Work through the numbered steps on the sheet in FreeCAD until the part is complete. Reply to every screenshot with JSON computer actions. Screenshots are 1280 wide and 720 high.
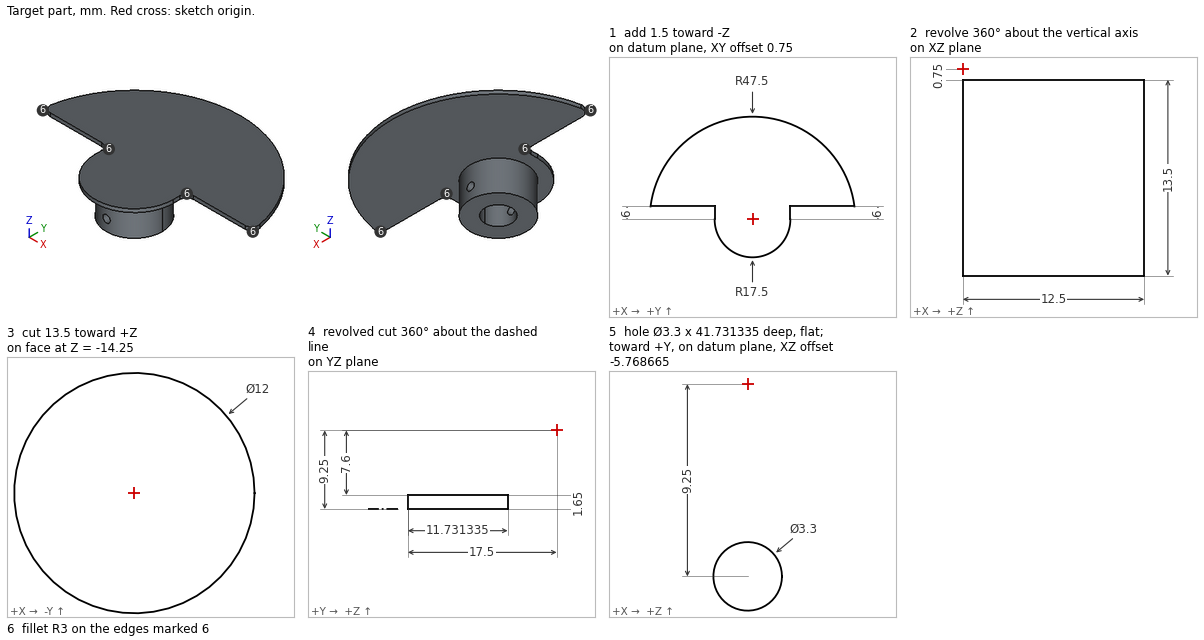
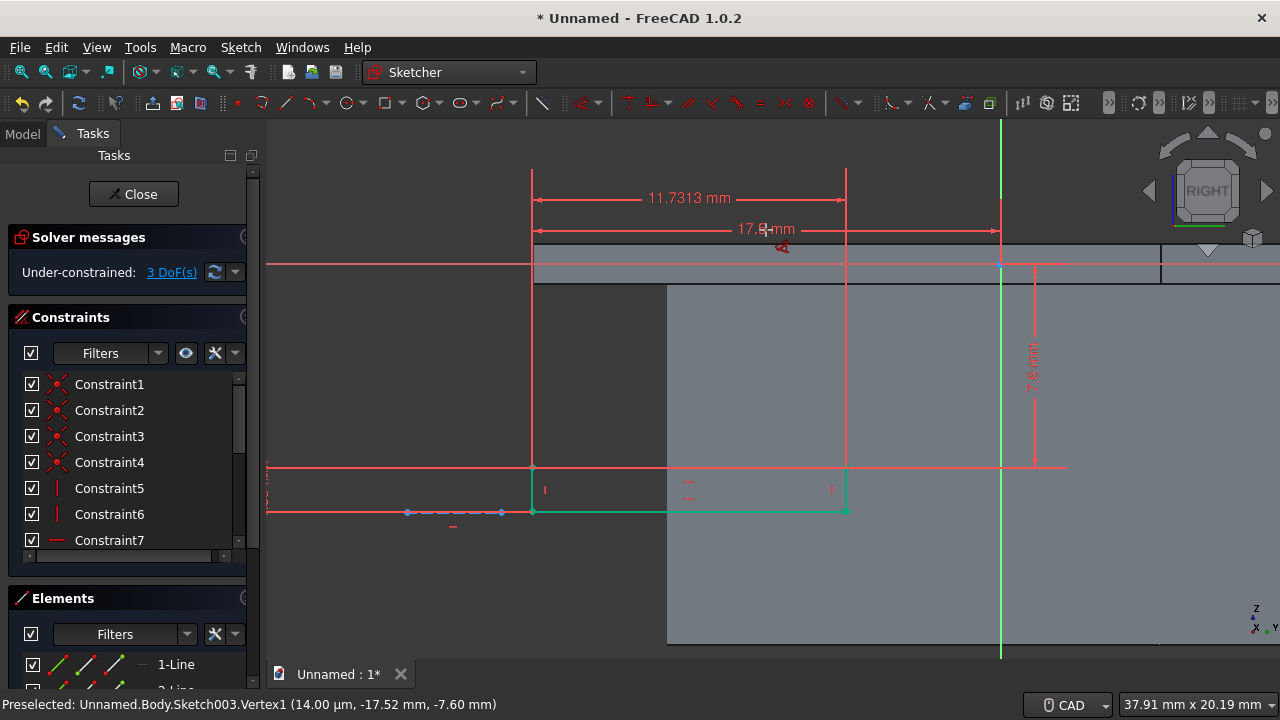
{"action": "left_click", "coordinate": [501, 513]}
{"action": "left_click", "coordinate": [1035, 389]}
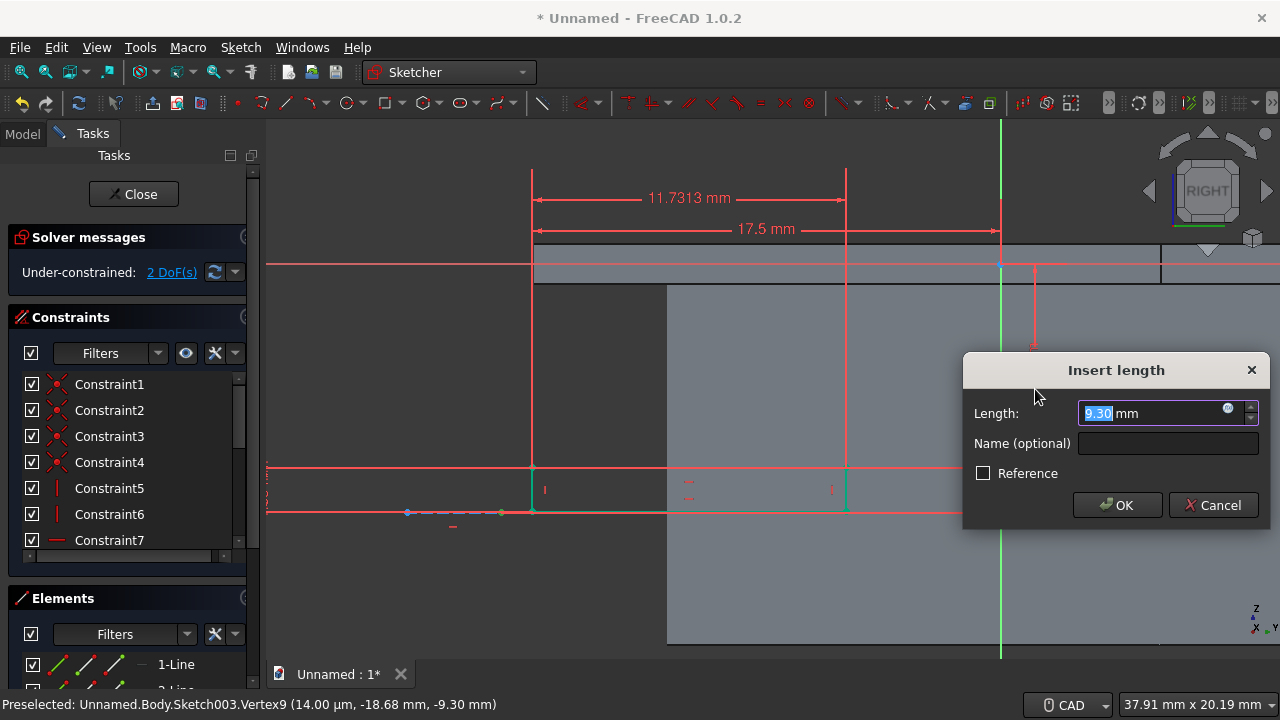
{"action": "type", "text": "9.25"}
{"action": "key", "text": "Return"}
{"action": "key", "text": "Escape"}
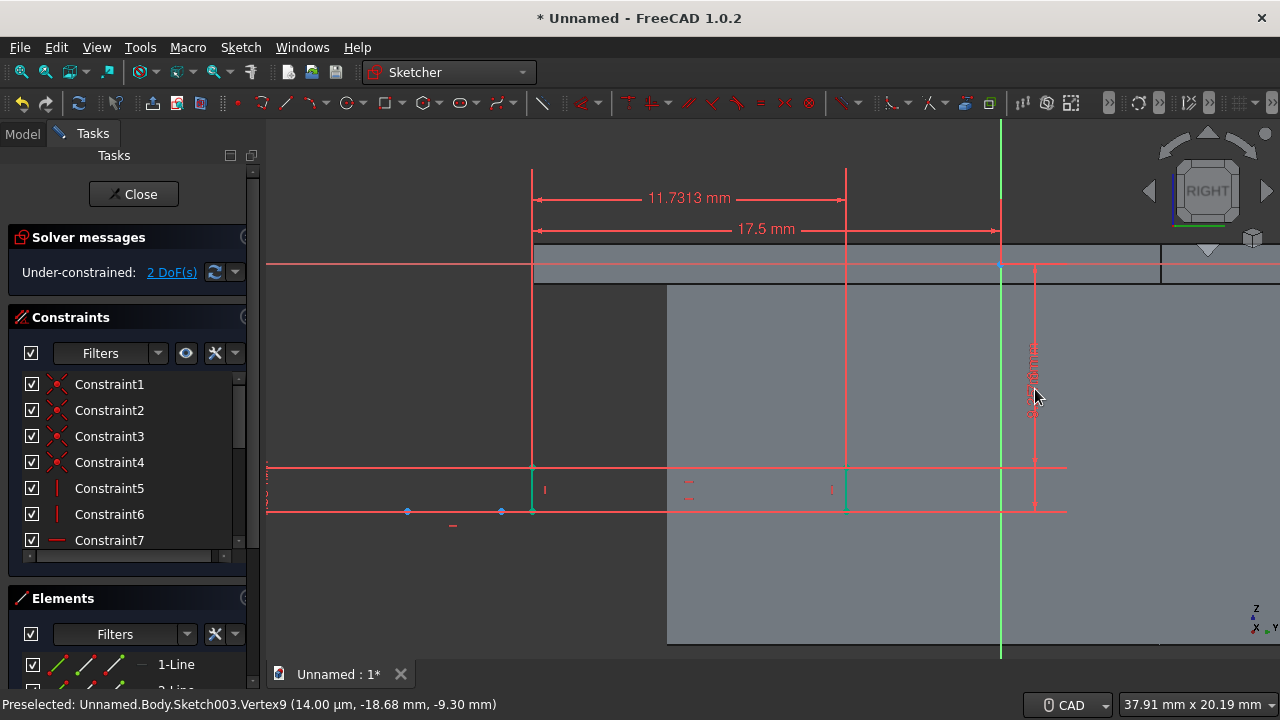
{"action": "left_click", "coordinate": [134, 194]}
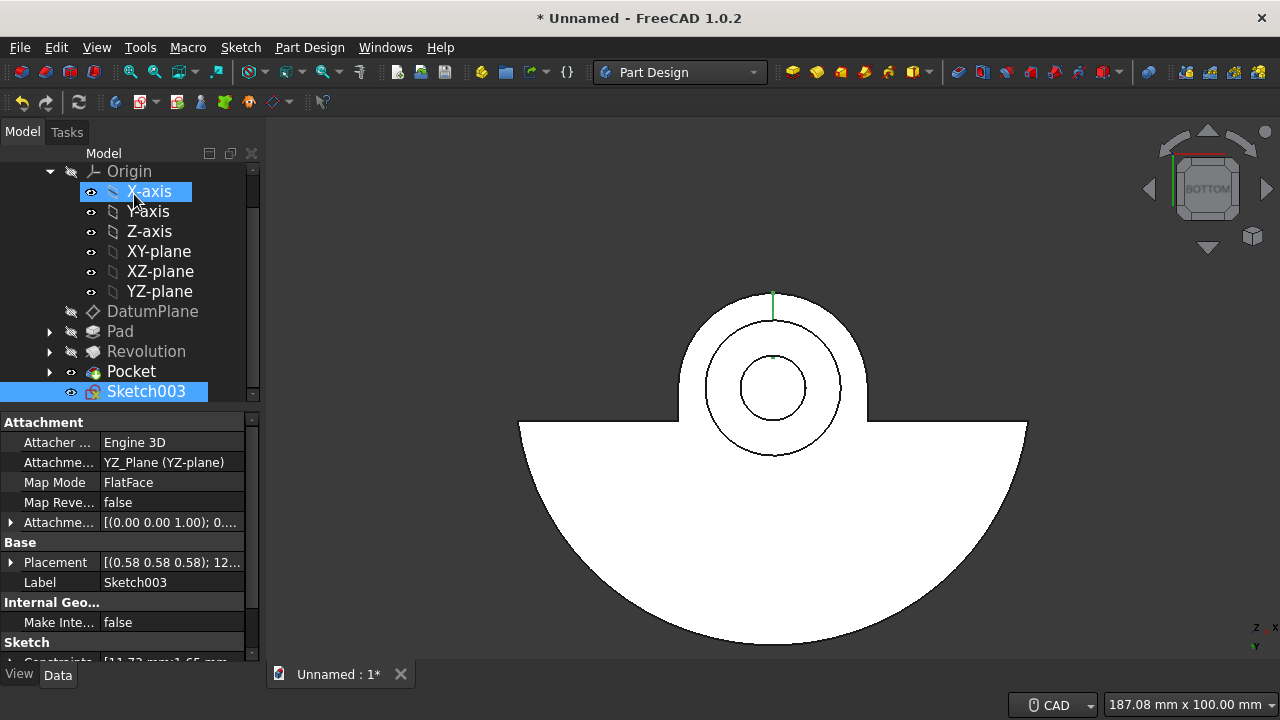
{"action": "left_click", "coordinate": [1008, 72]}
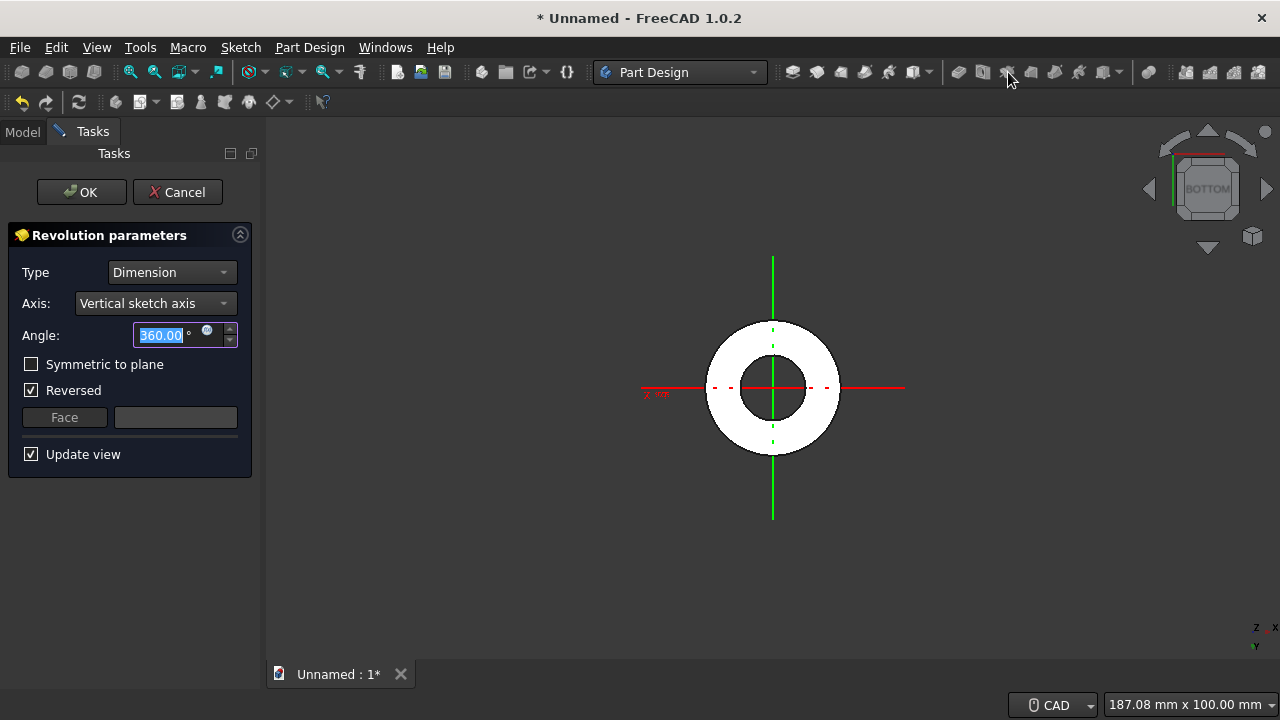
{"action": "left_click", "coordinate": [156, 304]}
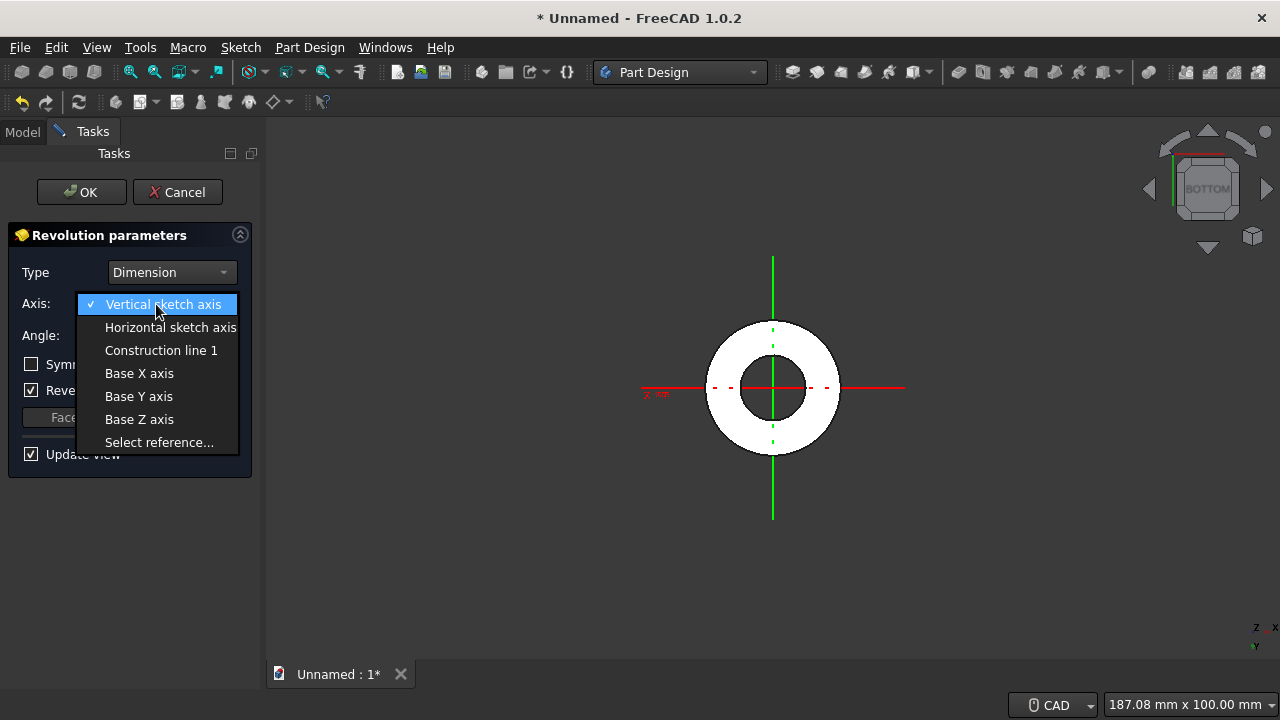
{"action": "left_click", "coordinate": [156, 350]}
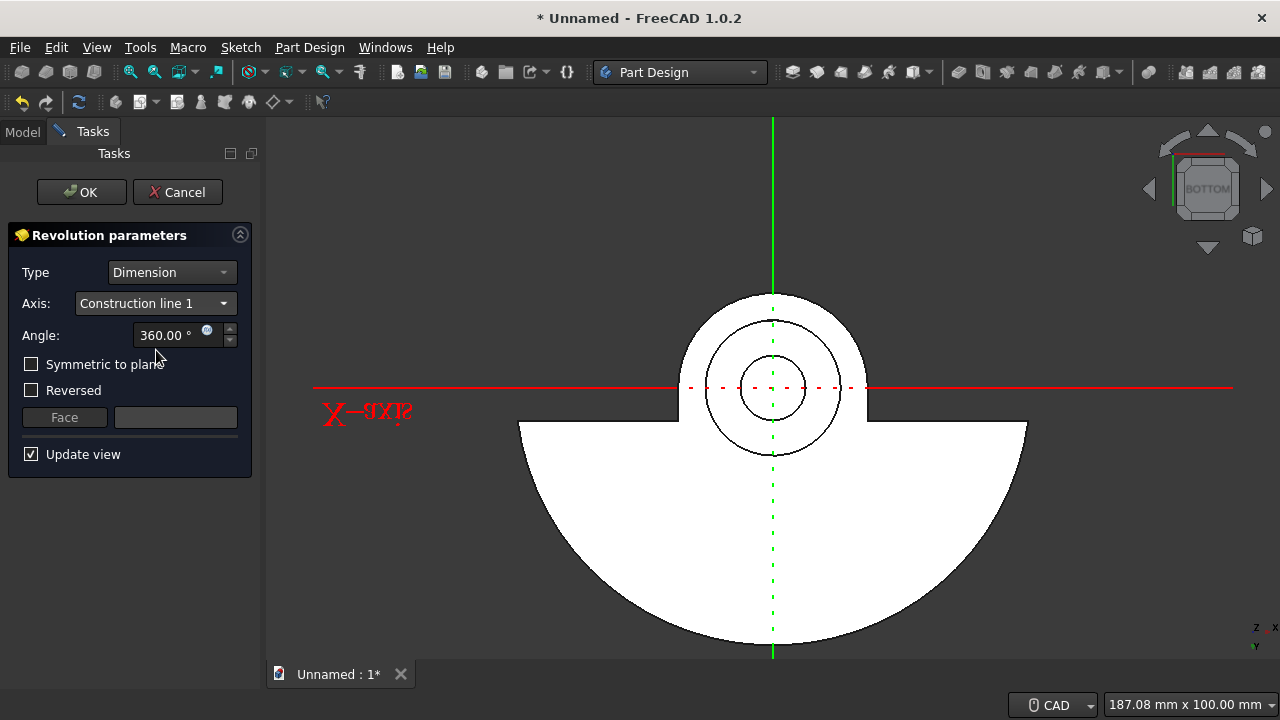
{"action": "left_click", "coordinate": [82, 192]}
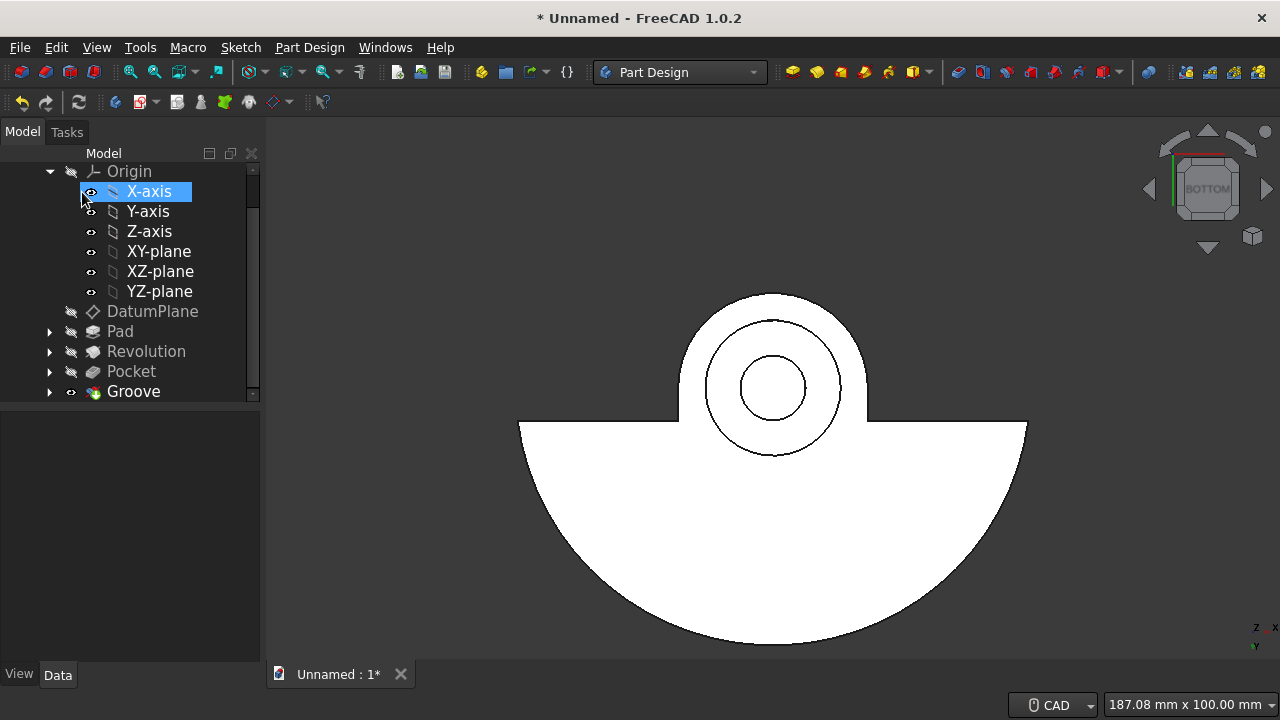
{"action": "left_click", "coordinate": [136, 272]}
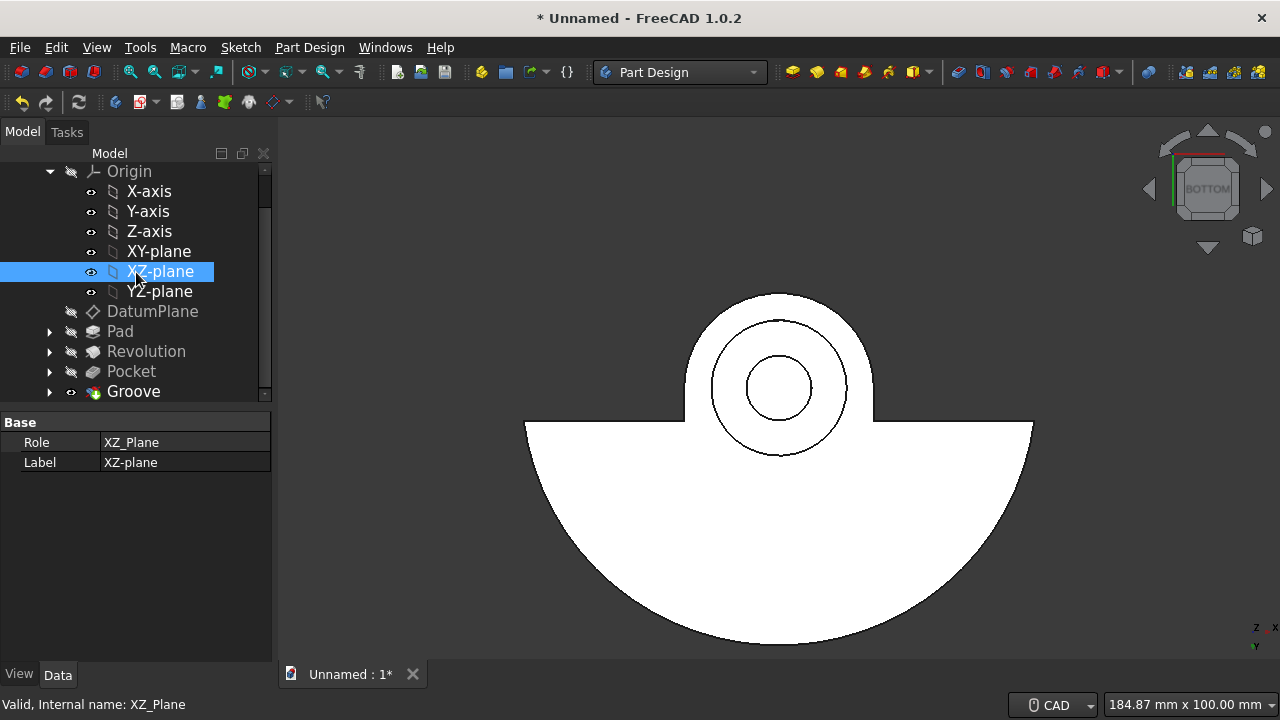
{"action": "left_click", "coordinate": [274, 102]}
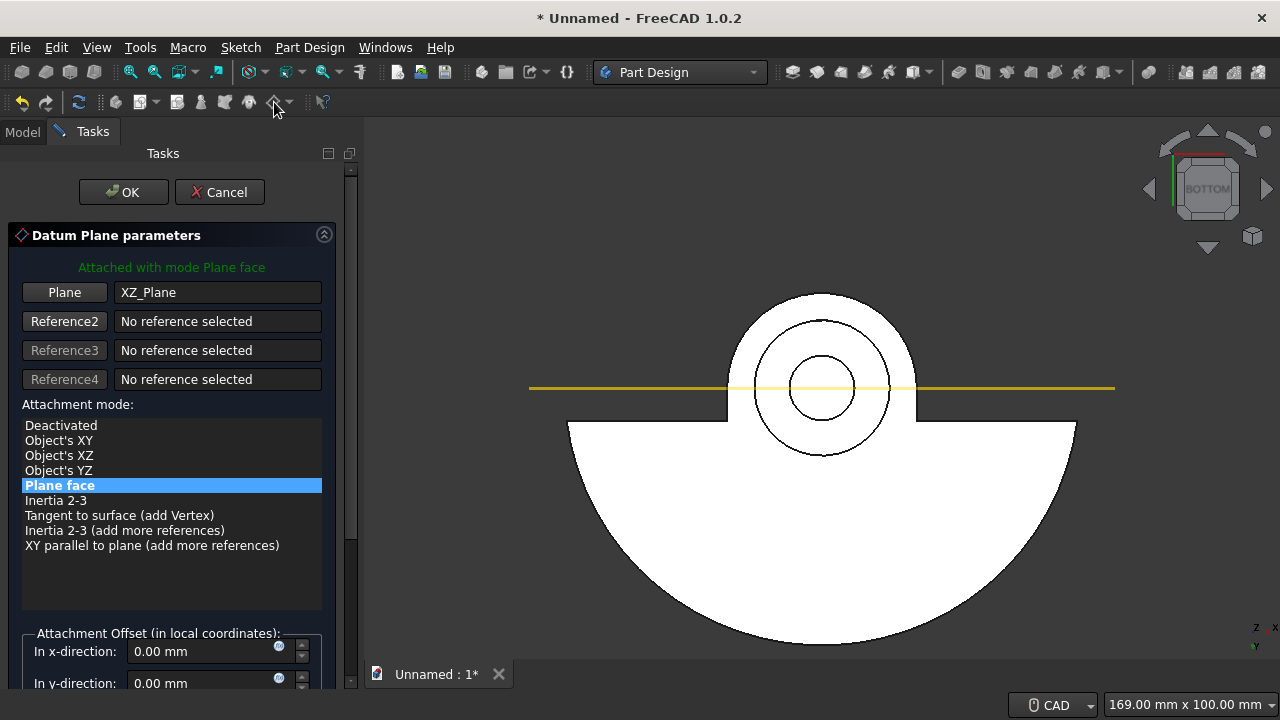
{"action": "scroll", "coordinate": [351, 426], "scroll_direction": "down", "scroll_amount": 2}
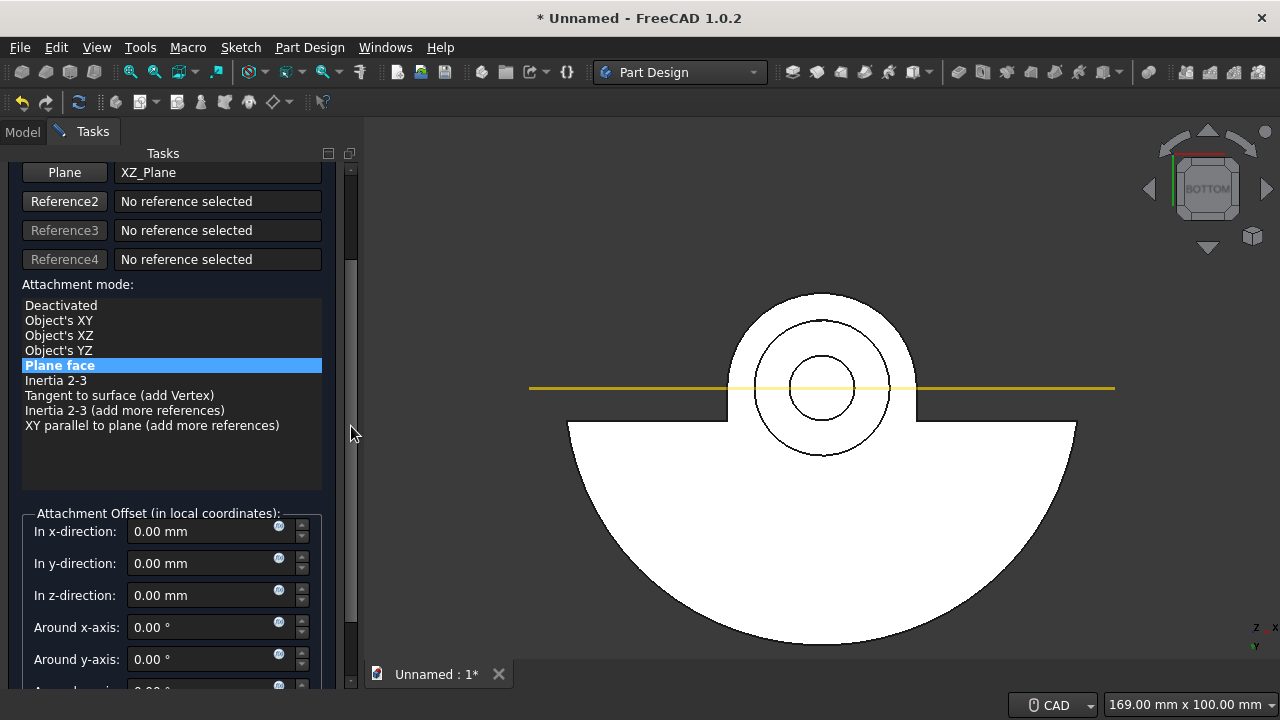
{"action": "triple_click", "coordinate": [210, 595]}